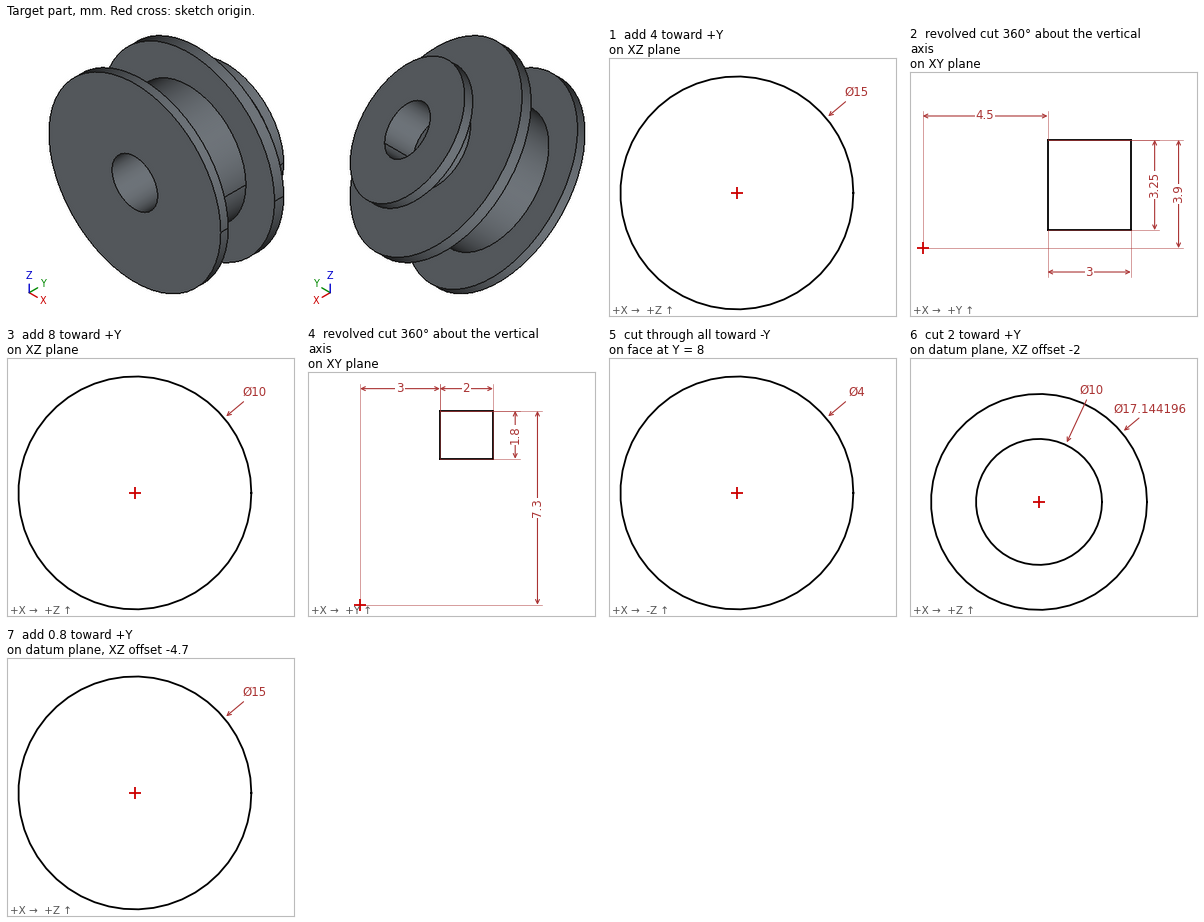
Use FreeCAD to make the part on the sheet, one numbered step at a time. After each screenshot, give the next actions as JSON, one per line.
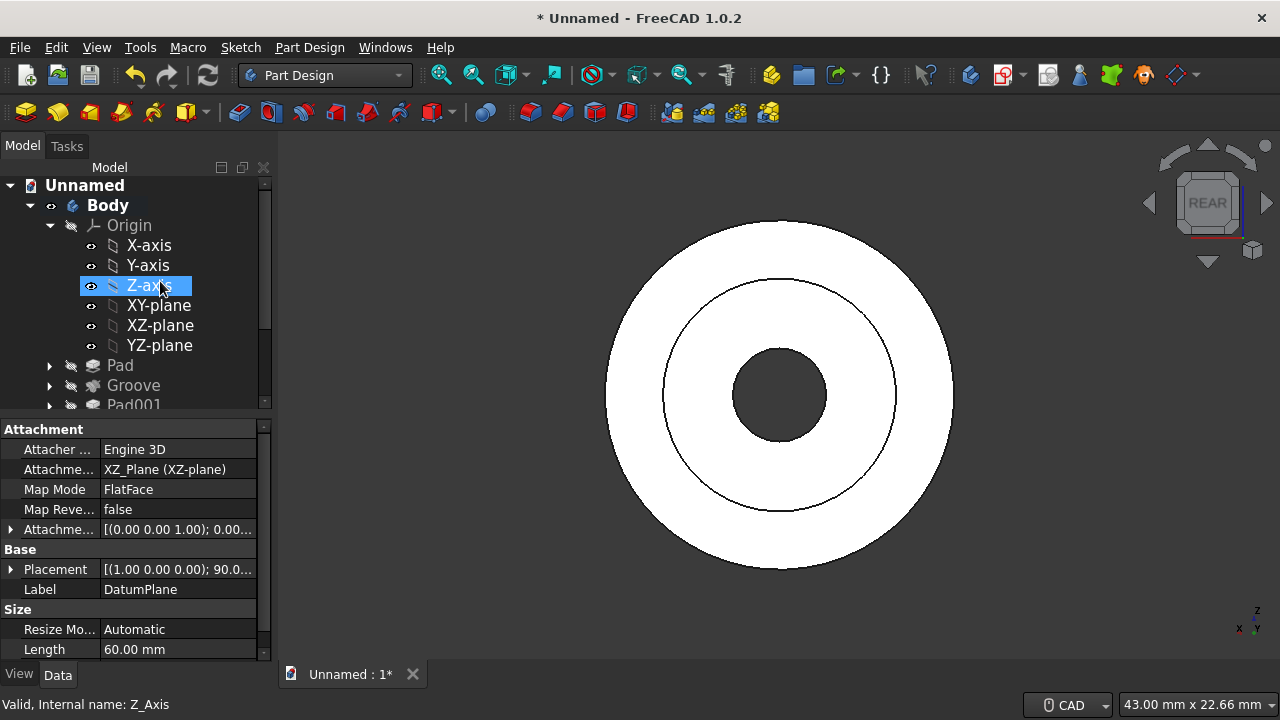
{"action": "left_click", "coordinate": [136, 326]}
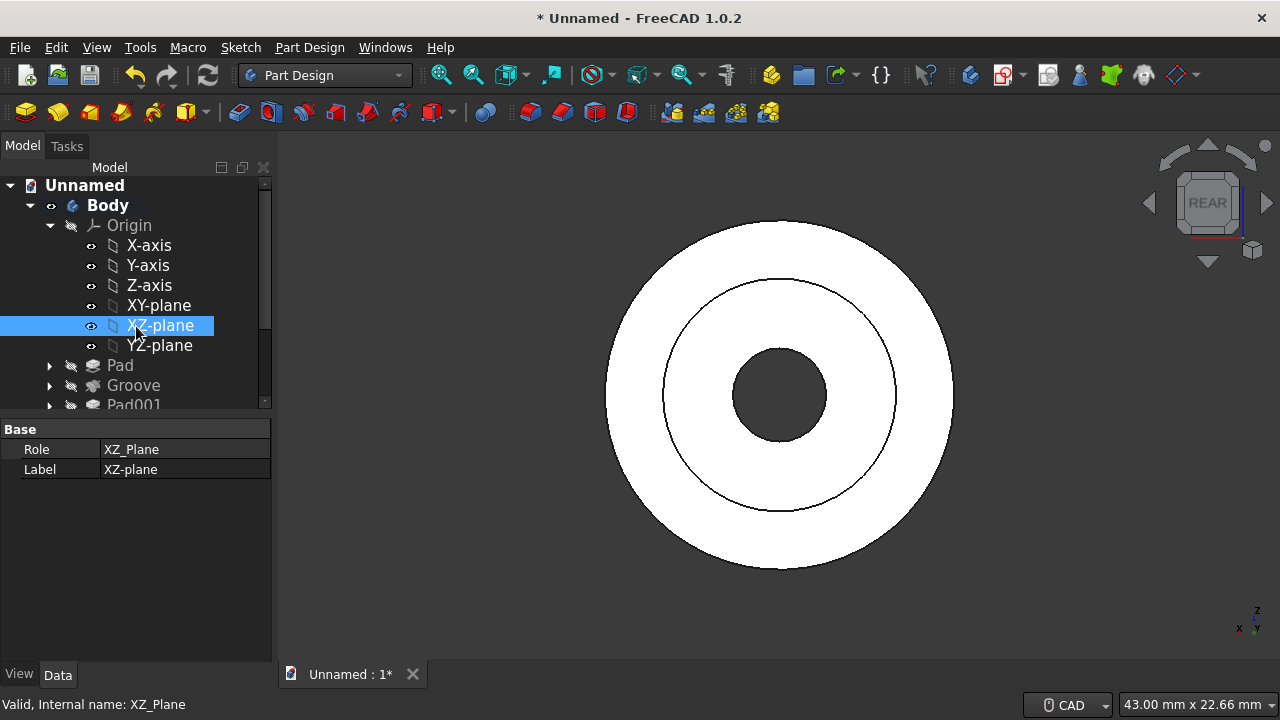
{"action": "left_click", "coordinate": [1176, 76]}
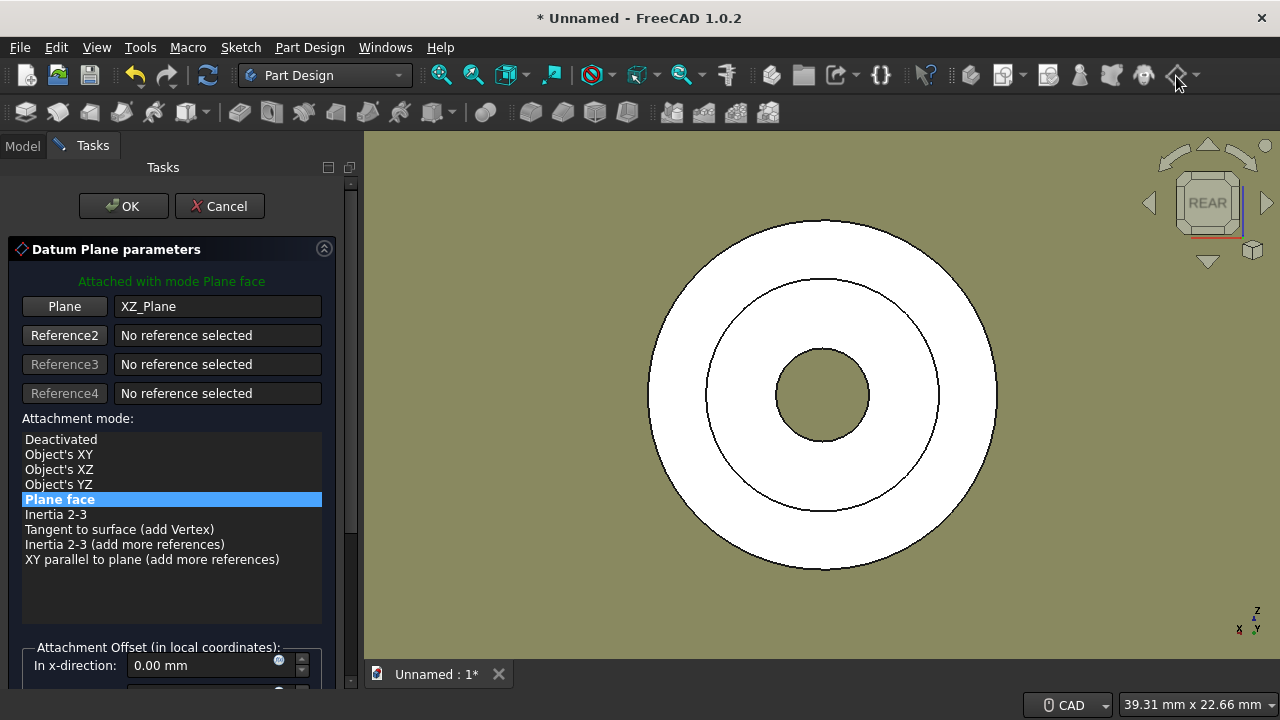
{"action": "scroll", "coordinate": [351, 432], "scroll_direction": "down", "scroll_amount": 2}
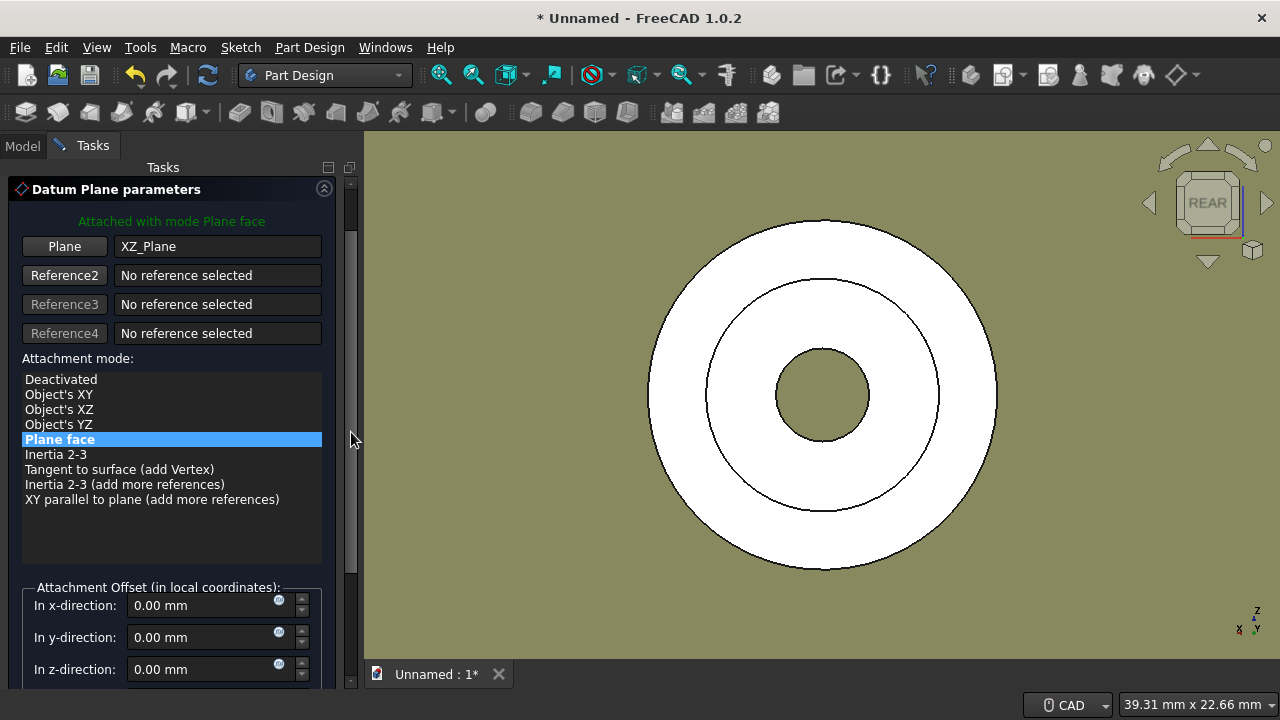
{"action": "triple_click", "coordinate": [210, 609]}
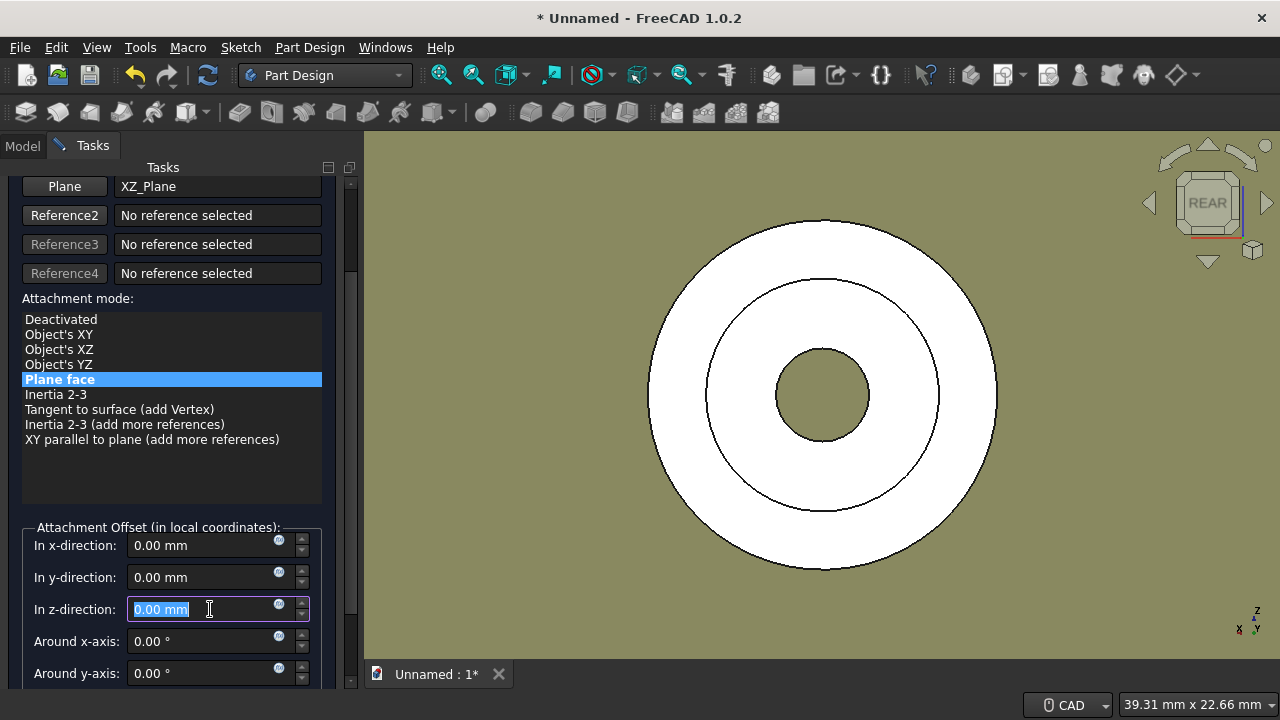
{"action": "type", "text": "-4.7"}
{"action": "key", "text": "Tab"}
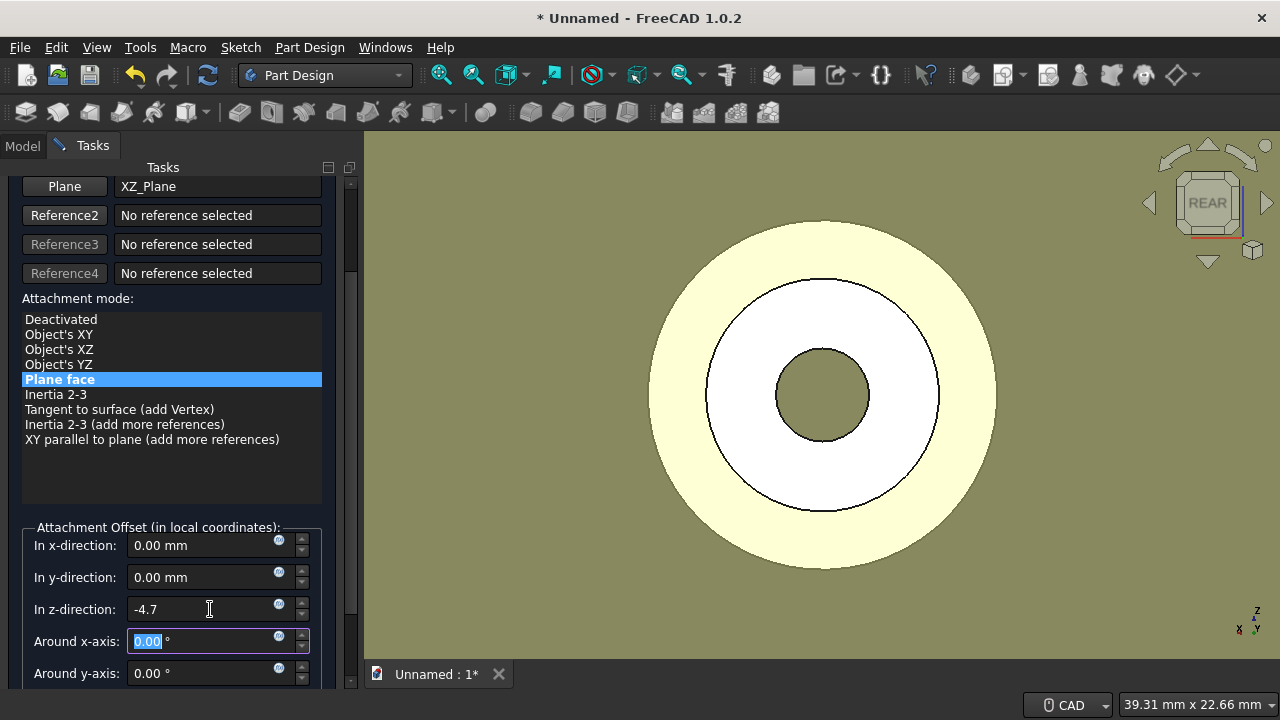
{"action": "scroll", "coordinate": [351, 432], "scroll_direction": "up", "scroll_amount": 3}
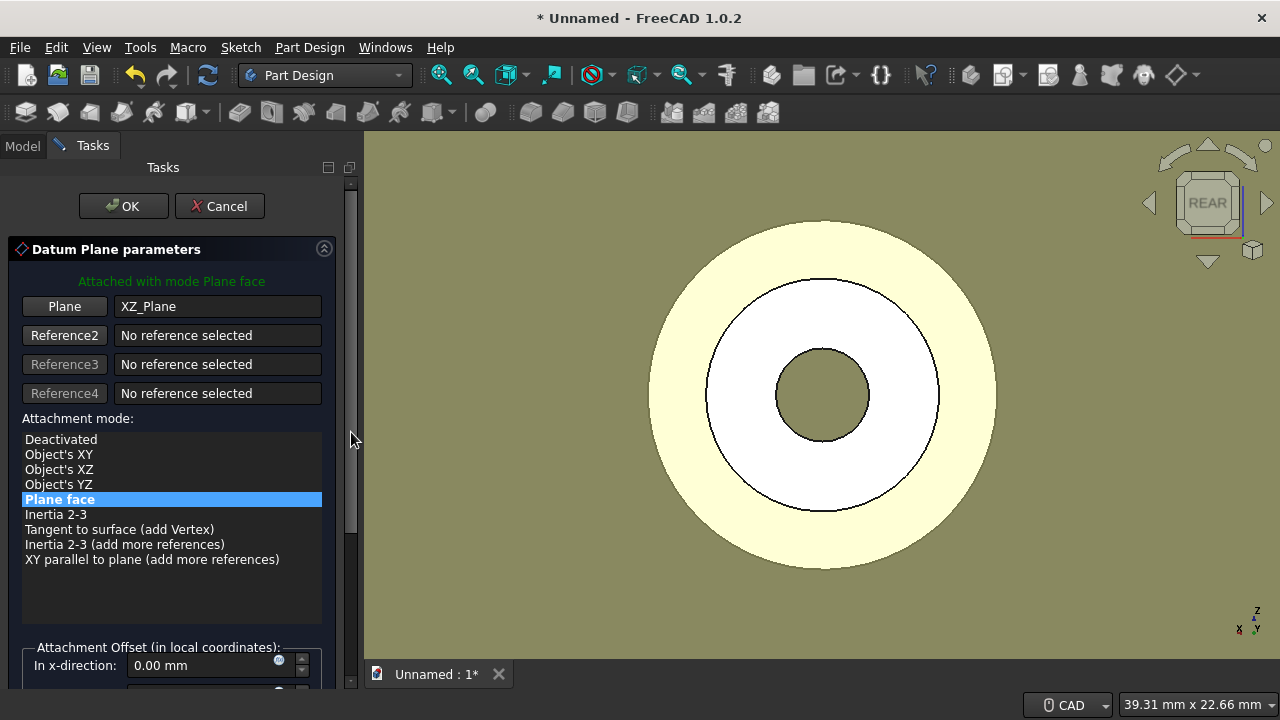
{"action": "left_click", "coordinate": [124, 206]}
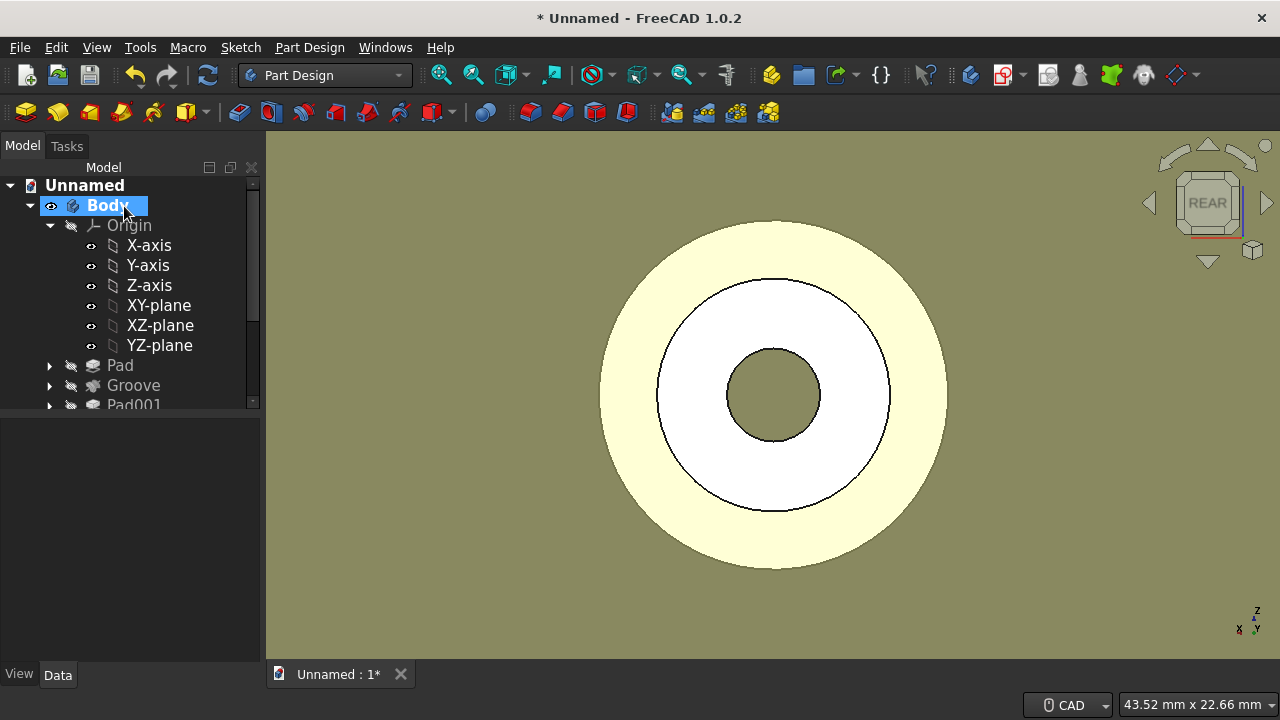
{"action": "scroll", "coordinate": [100, 301], "scroll_direction": "down", "scroll_amount": 3}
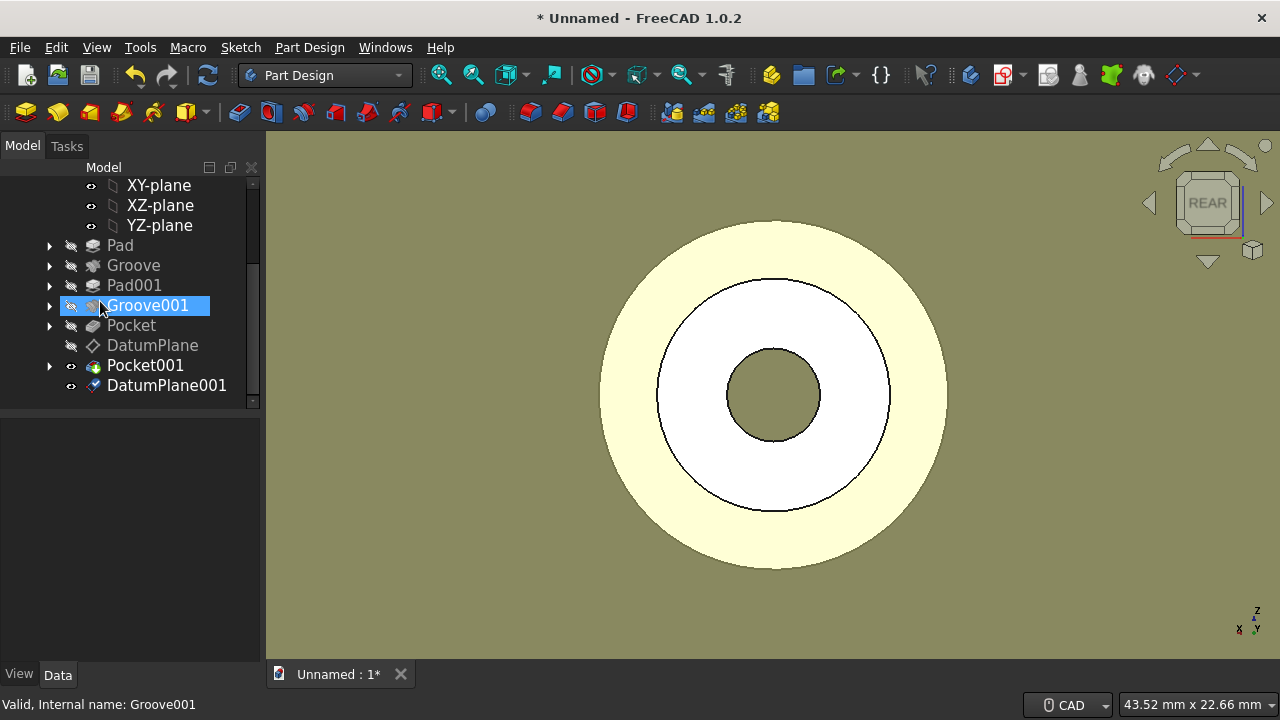
{"action": "left_click", "coordinate": [116, 386]}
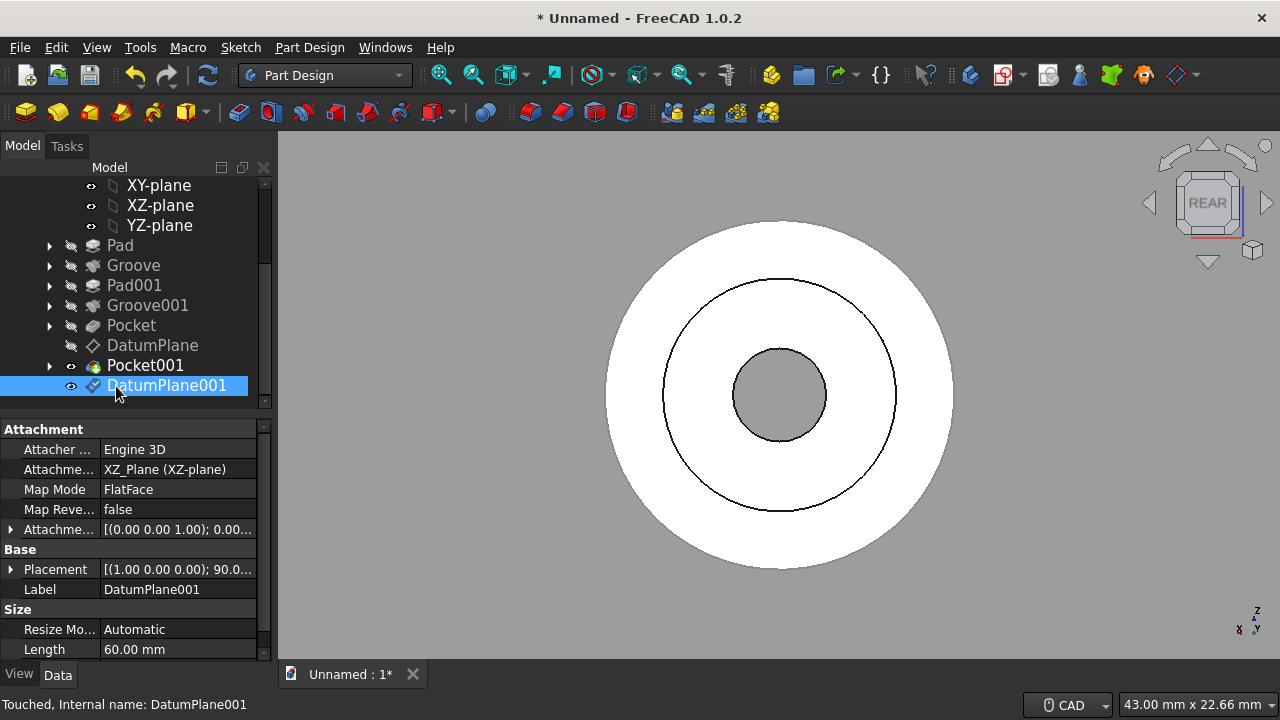
{"action": "left_click", "coordinate": [1004, 76]}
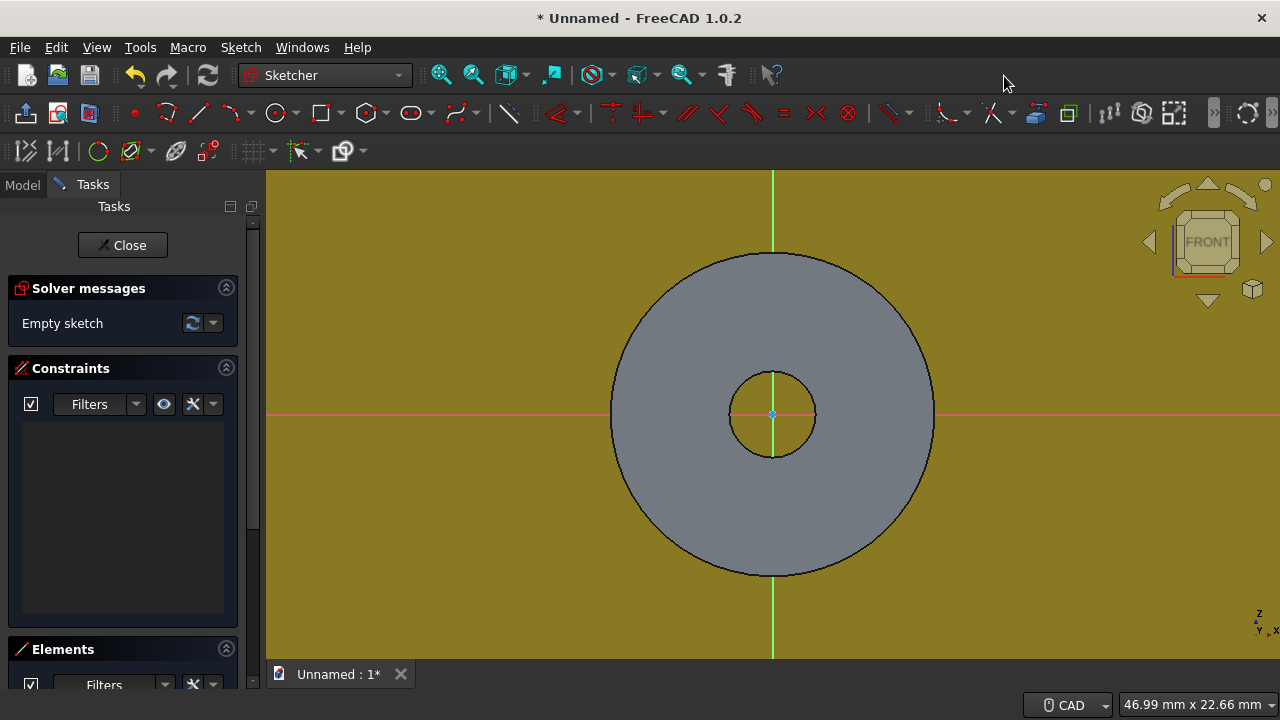
{"action": "key", "text": "q s"}